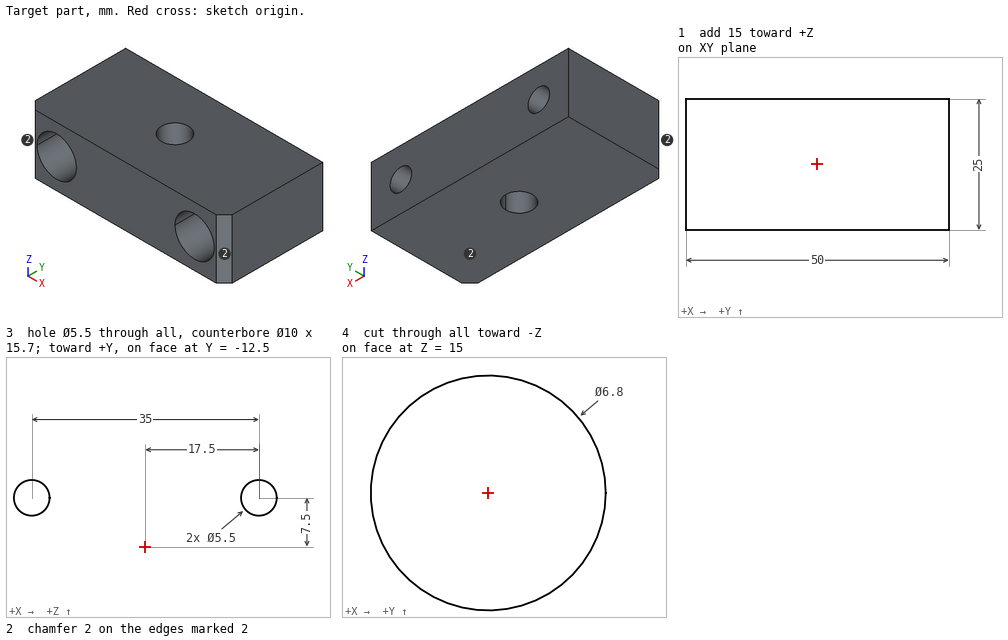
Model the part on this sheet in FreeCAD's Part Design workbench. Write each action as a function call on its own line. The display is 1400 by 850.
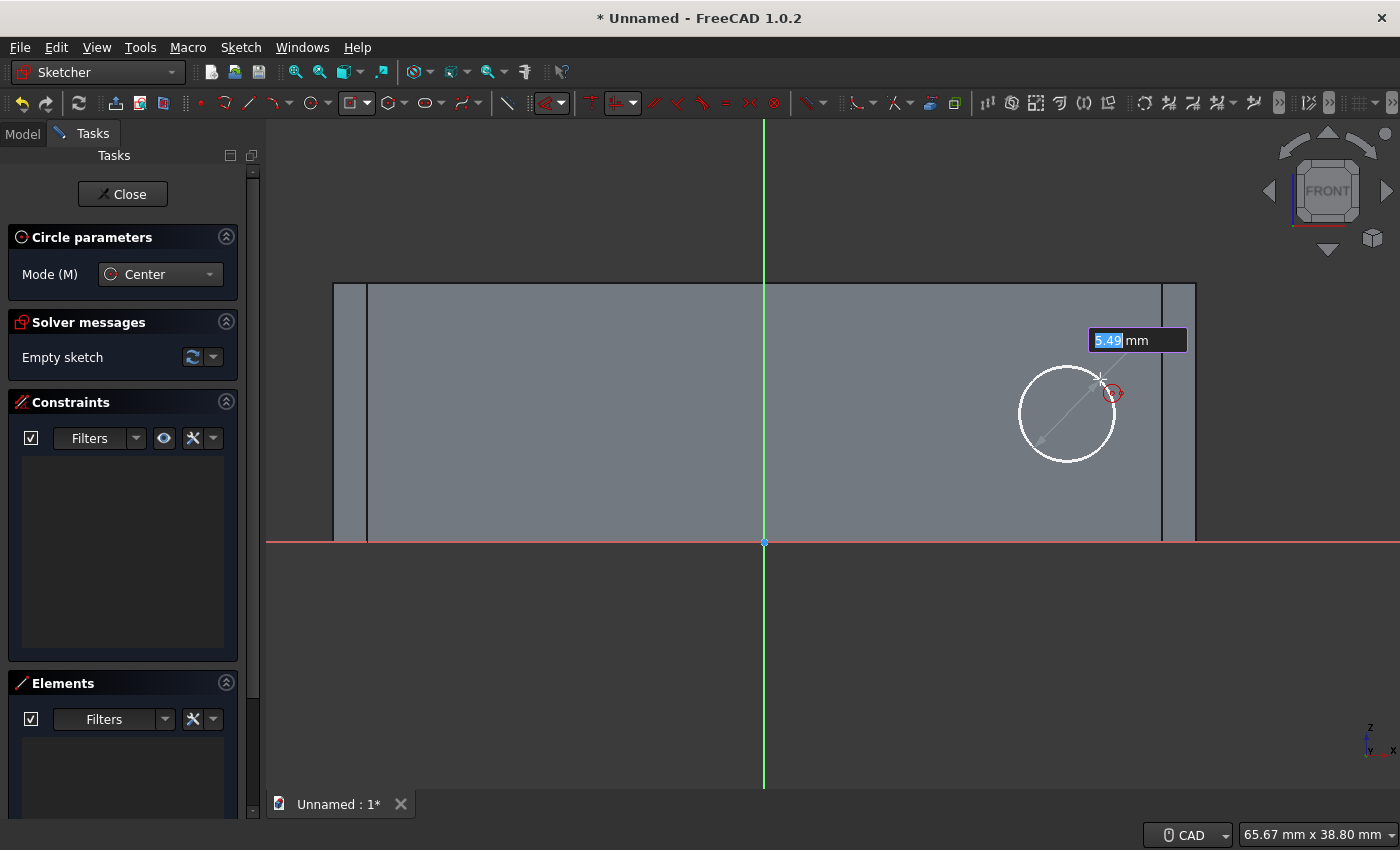
text(5.5)
key(Return)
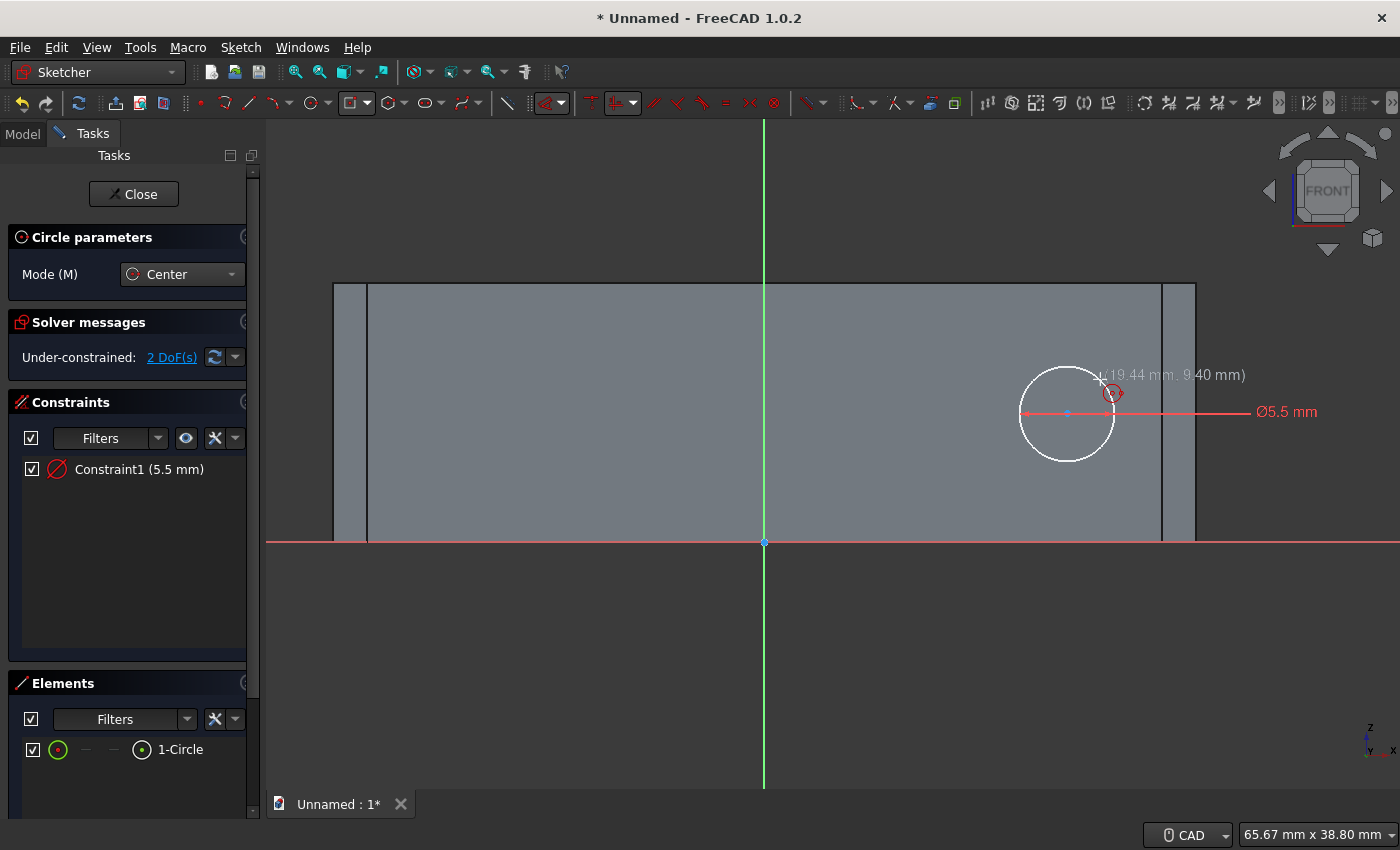
click(462, 413)
move(496, 379)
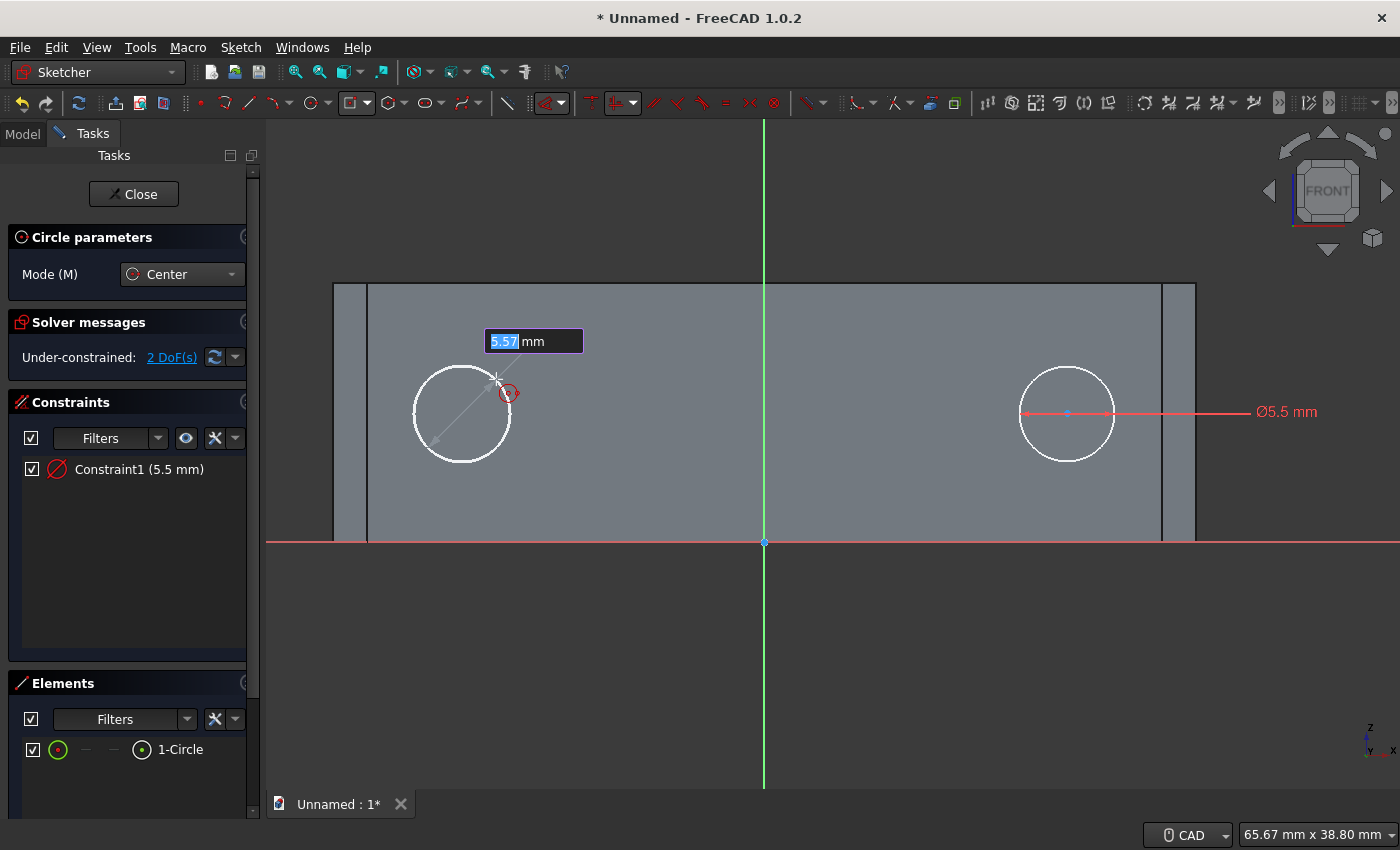
text(5.5)
key(Return)
key(Escape)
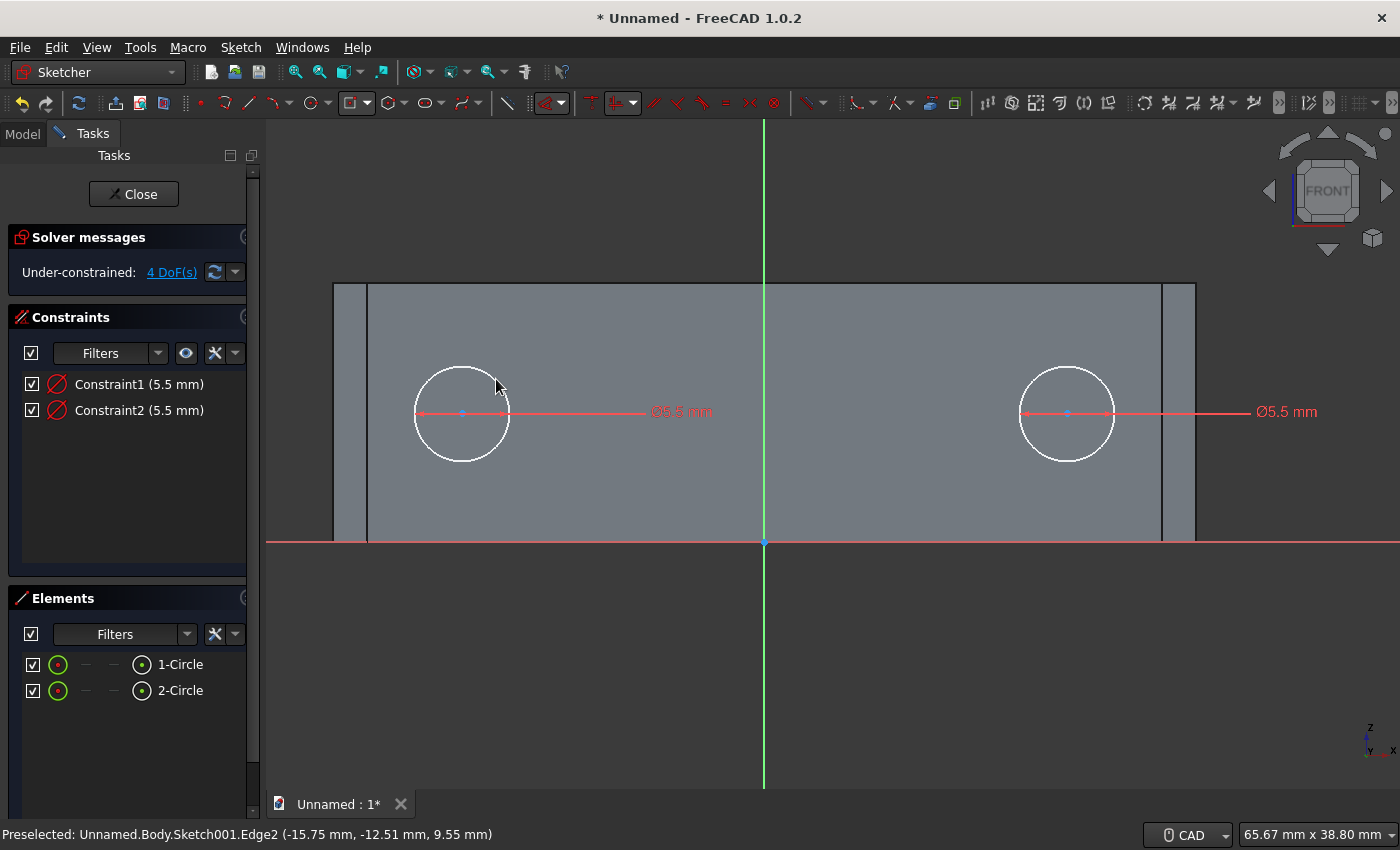
click(1067, 414)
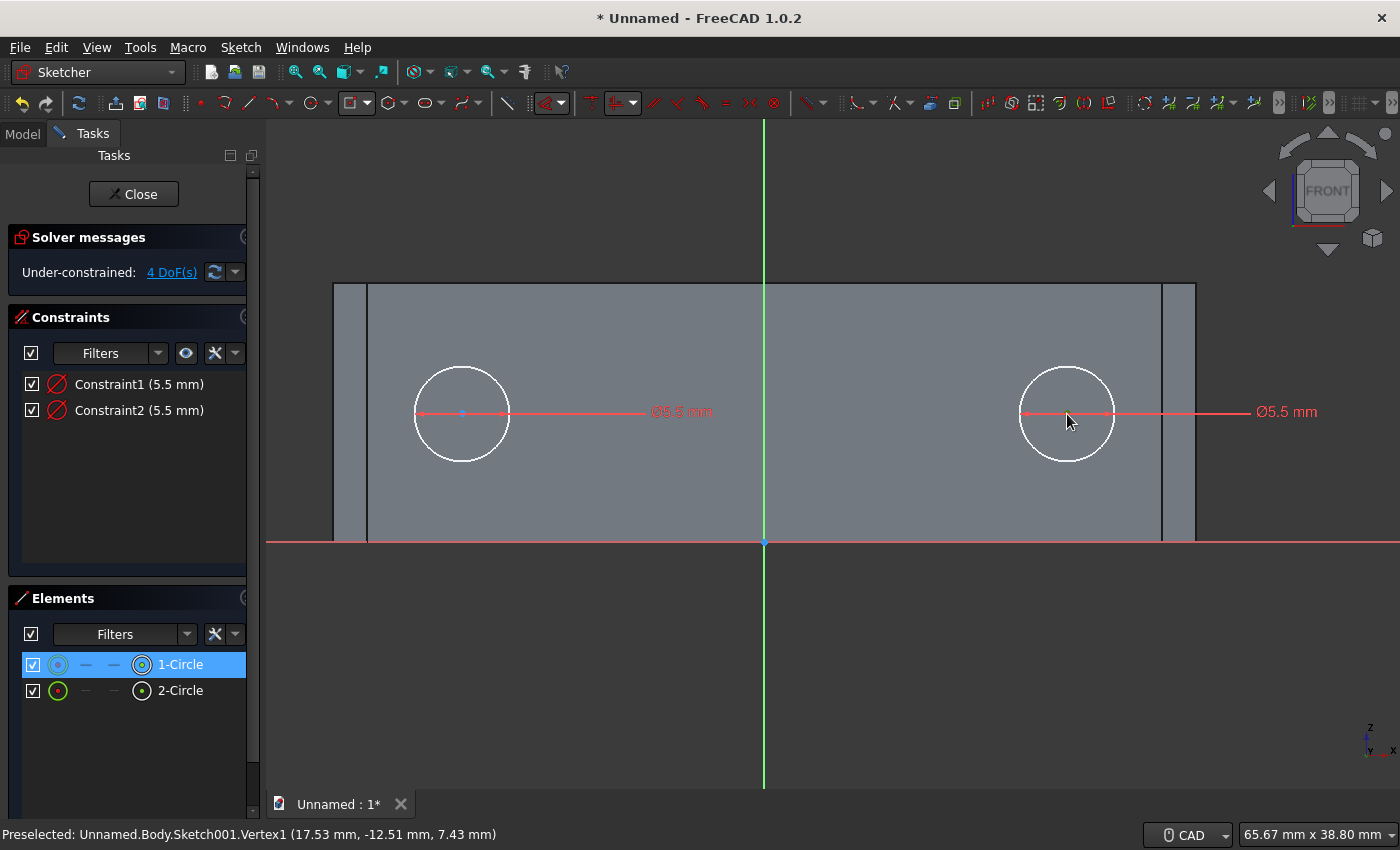
click(462, 414)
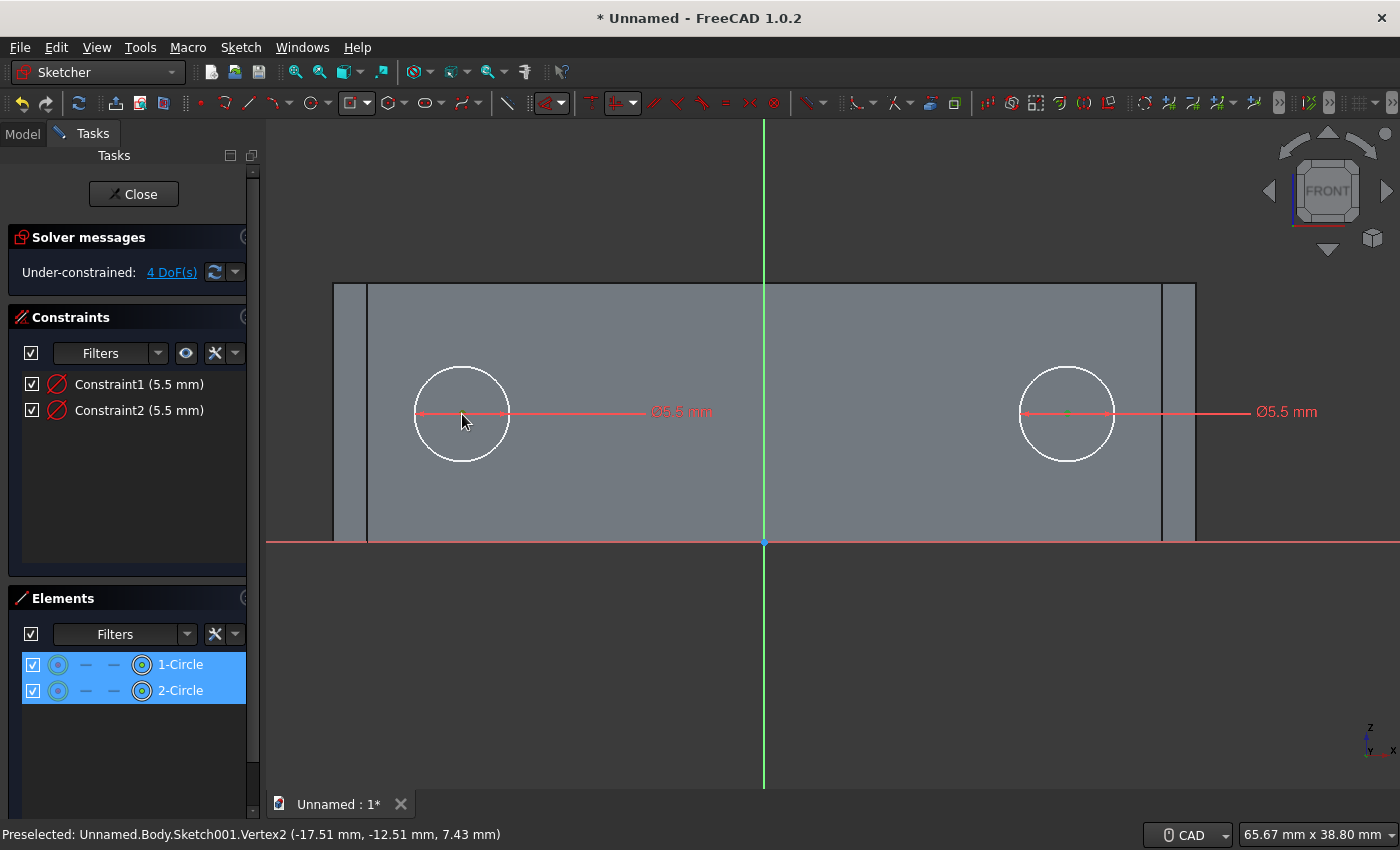
key(h)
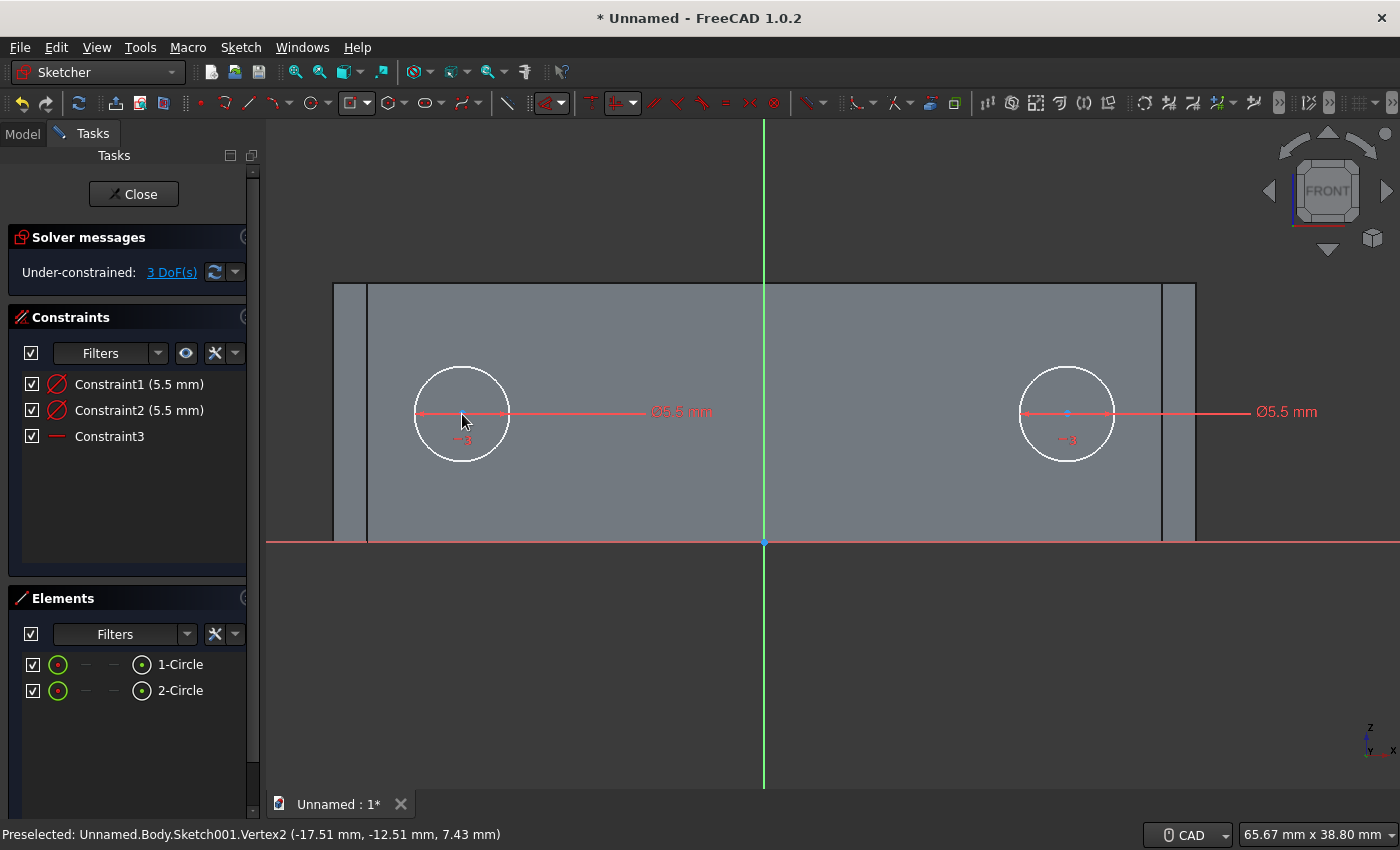
click(1067, 414)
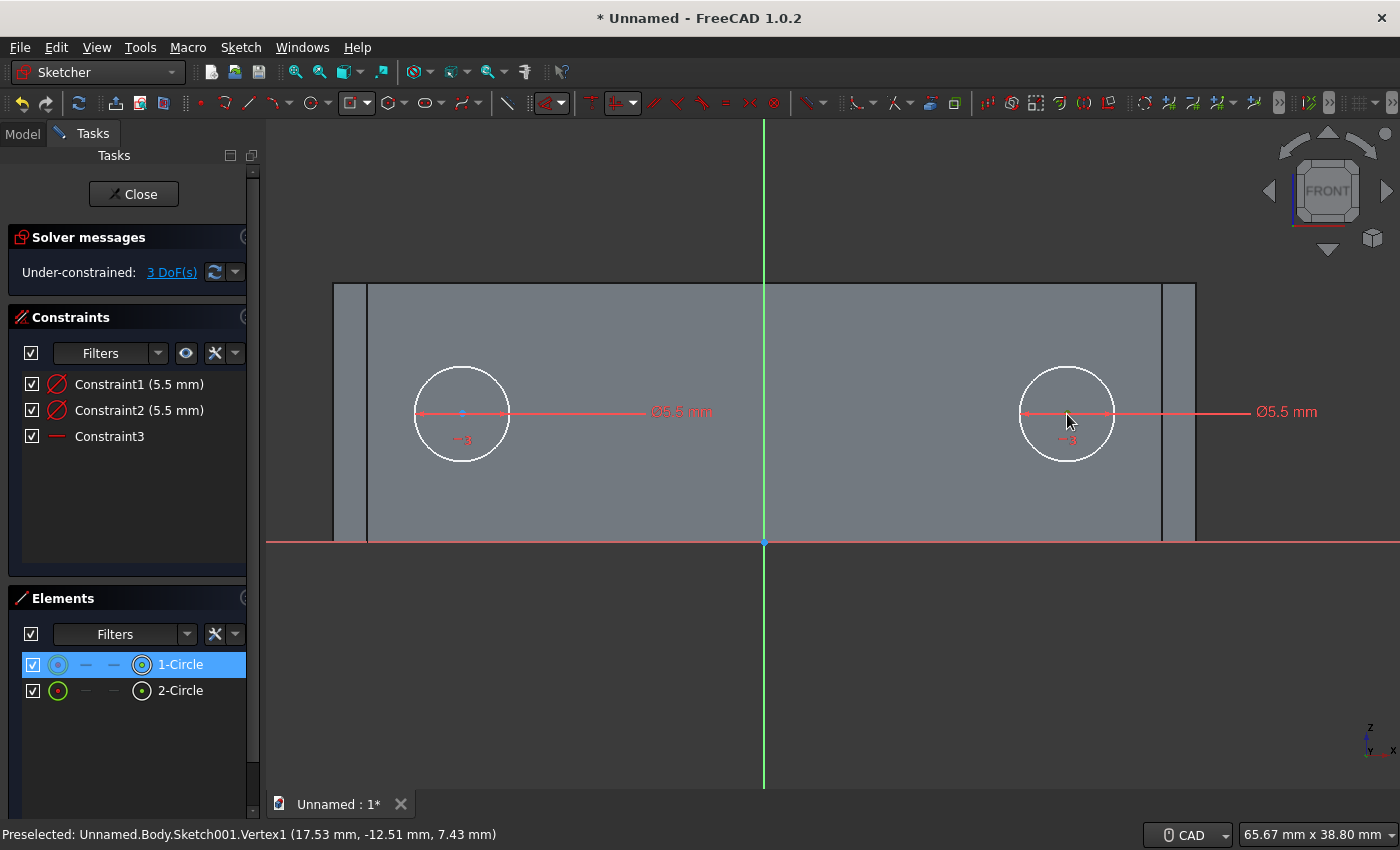
key(i)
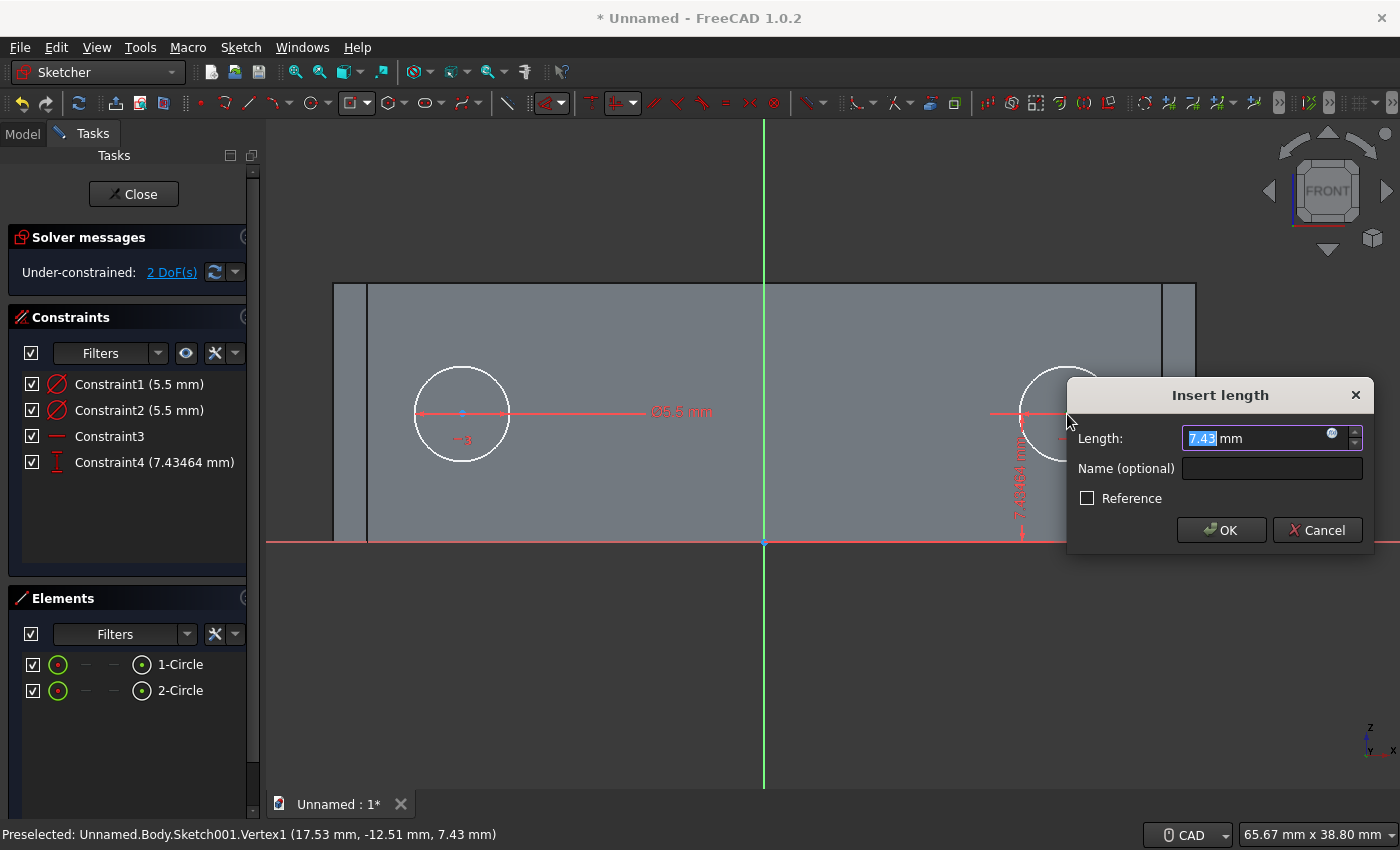
text(7.5)
key(Return)